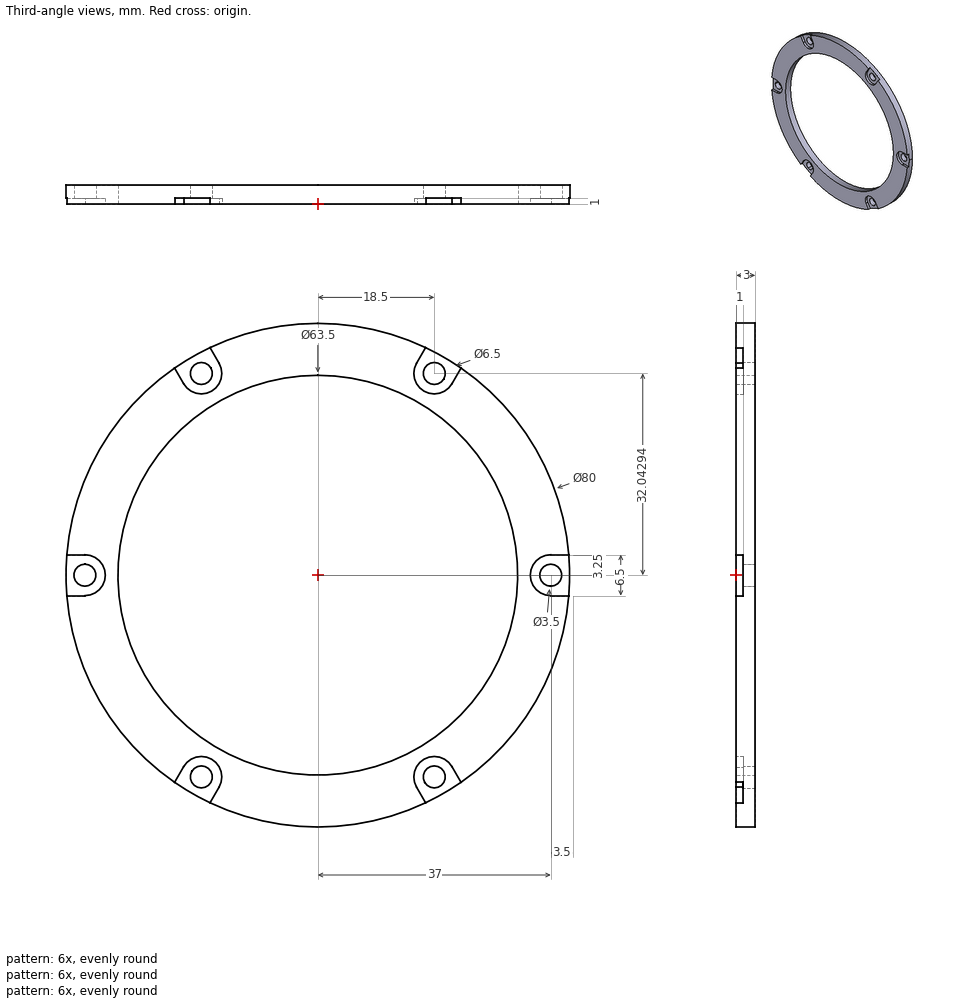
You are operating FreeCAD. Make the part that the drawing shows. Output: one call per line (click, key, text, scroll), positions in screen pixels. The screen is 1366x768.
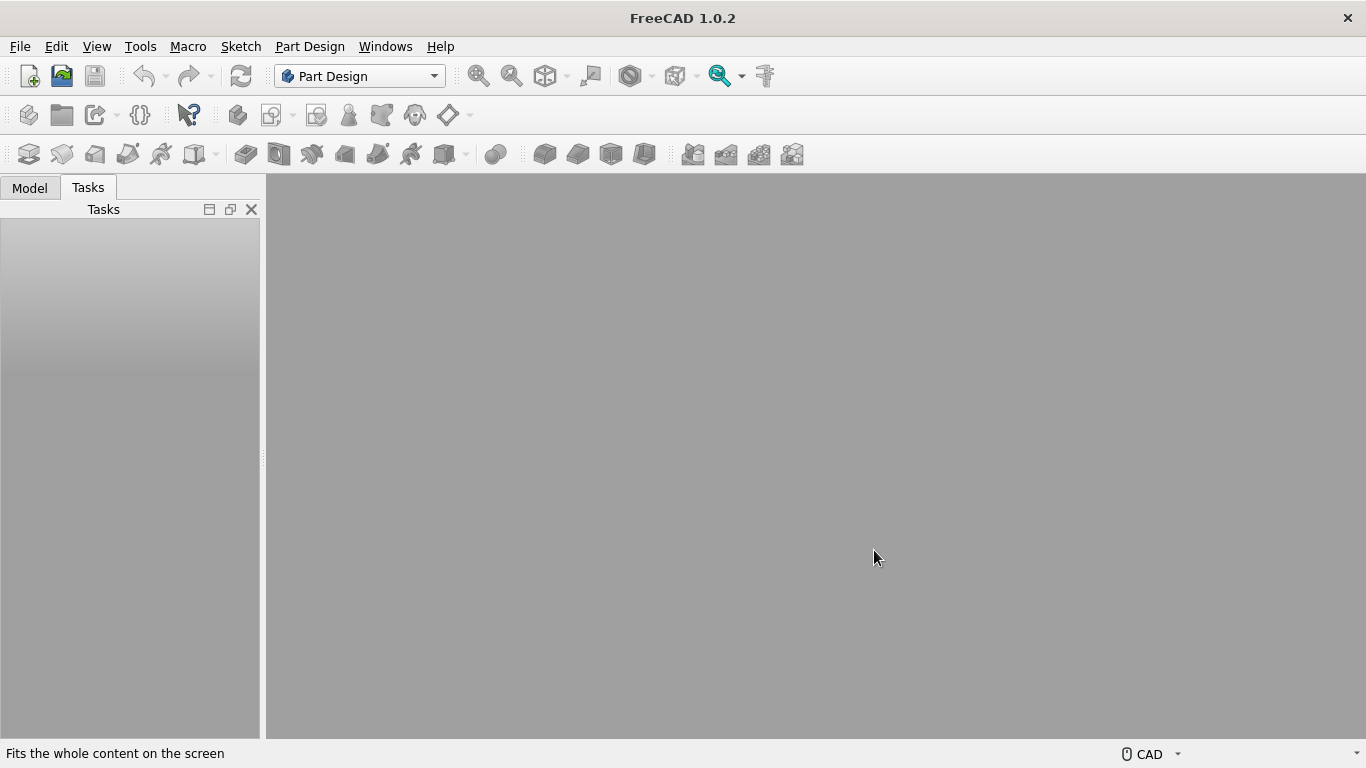
click(29, 76)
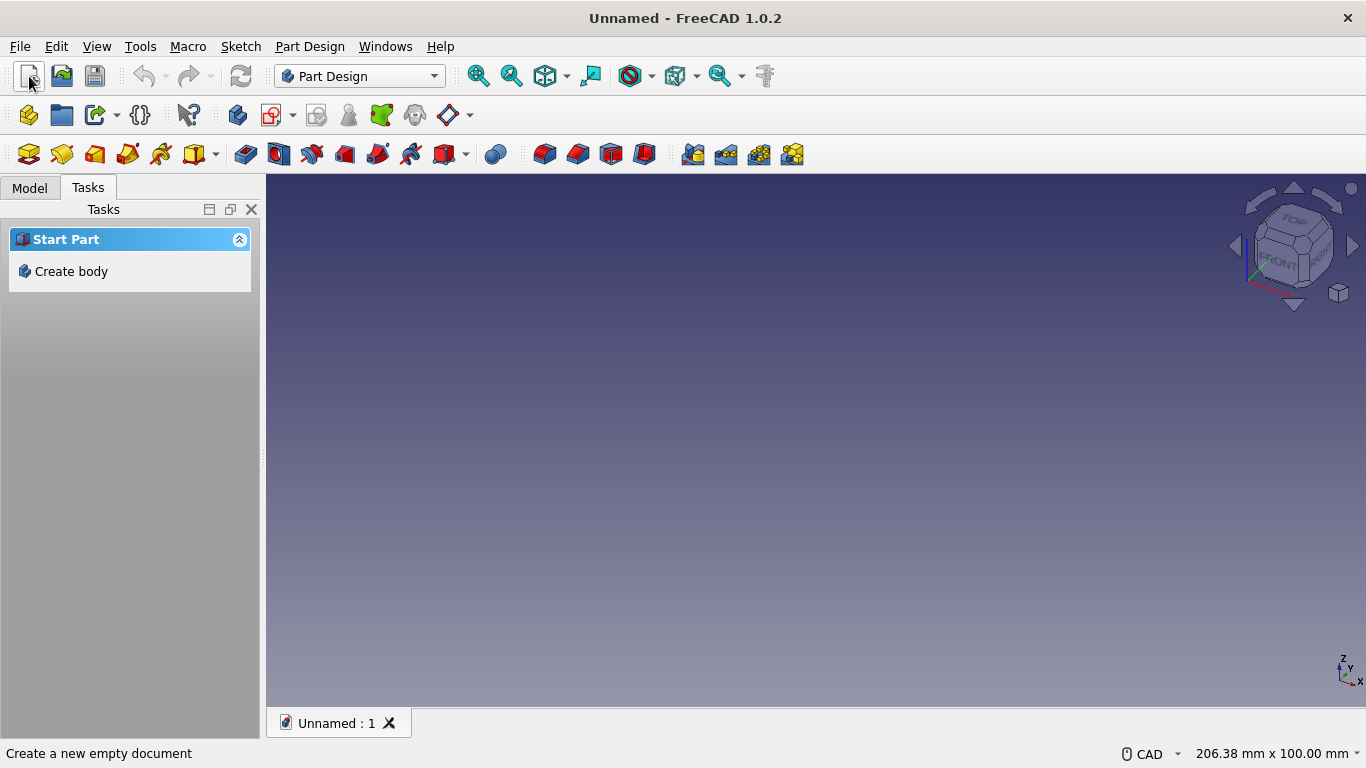
click(270, 116)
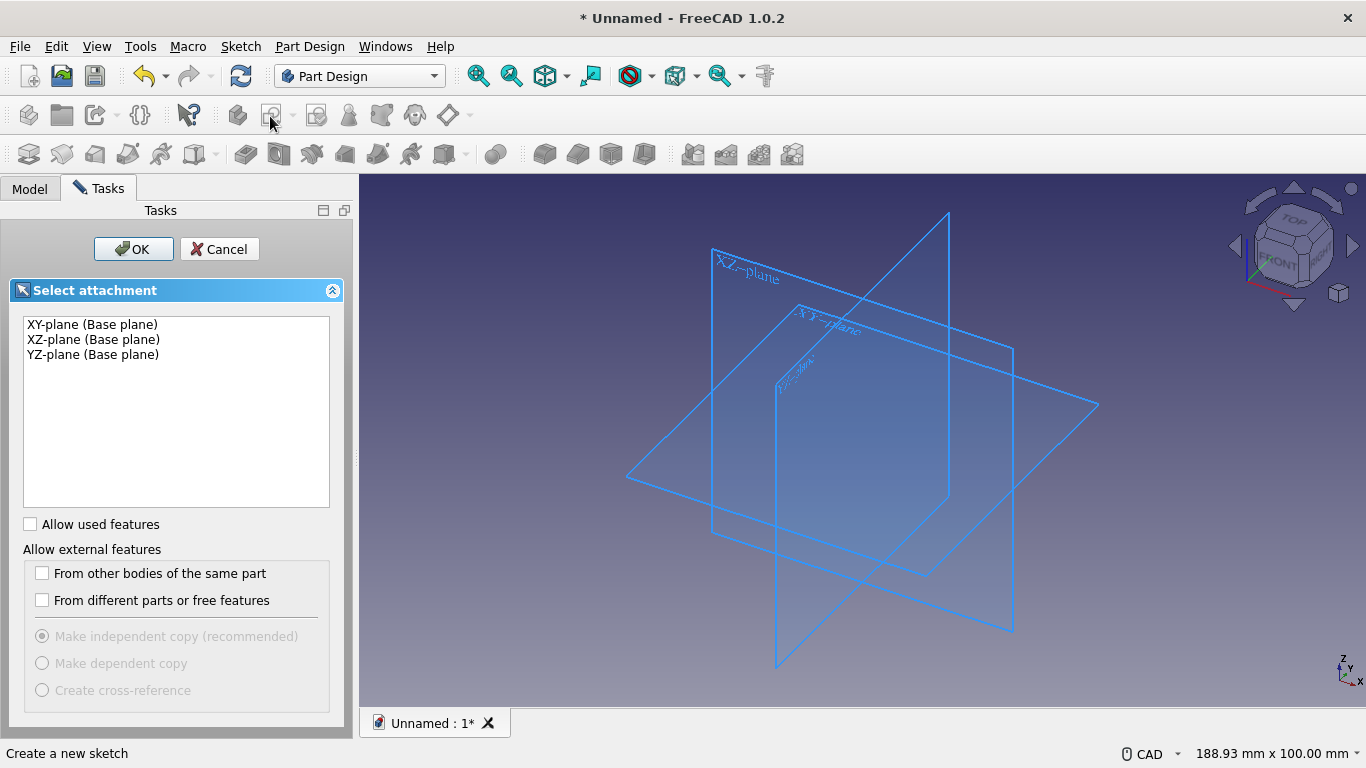
click(84, 340)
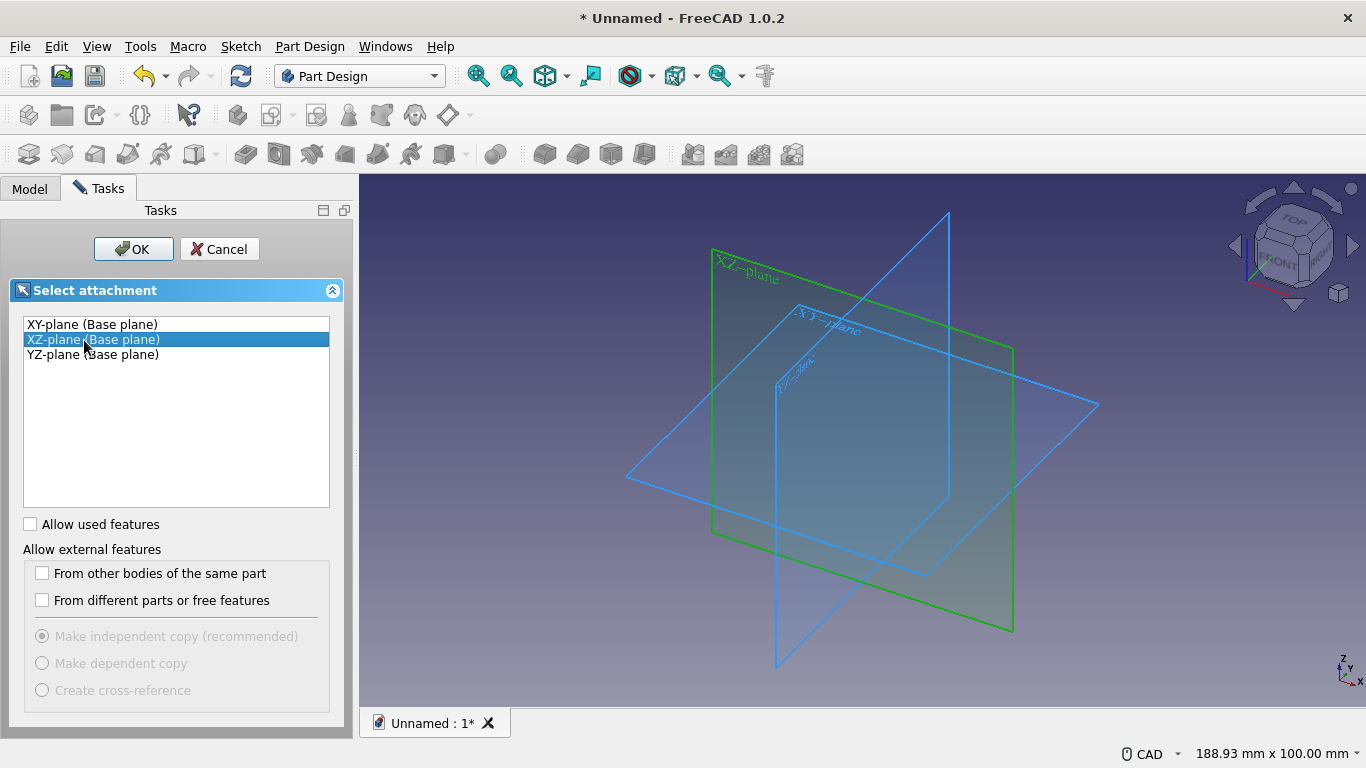
click(134, 249)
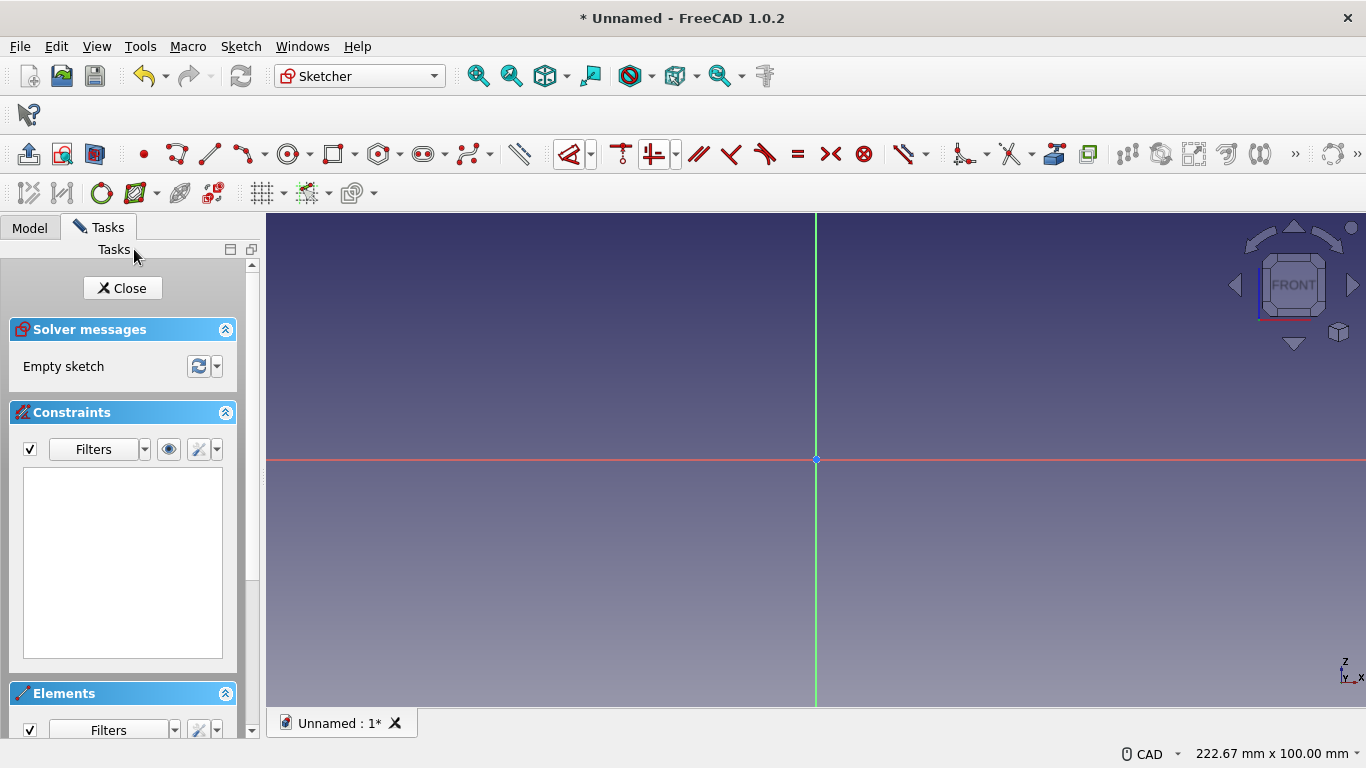
scroll(438, 460, down, 1)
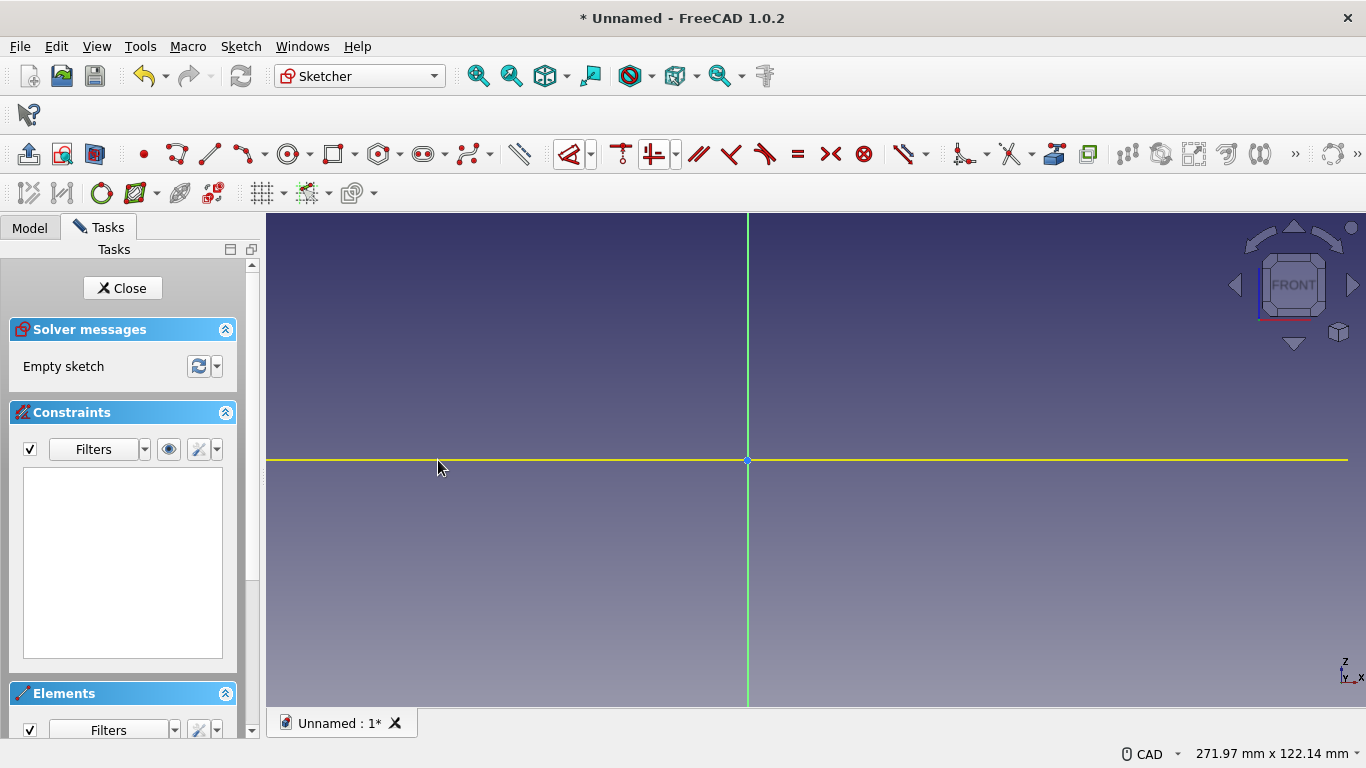
click(288, 154)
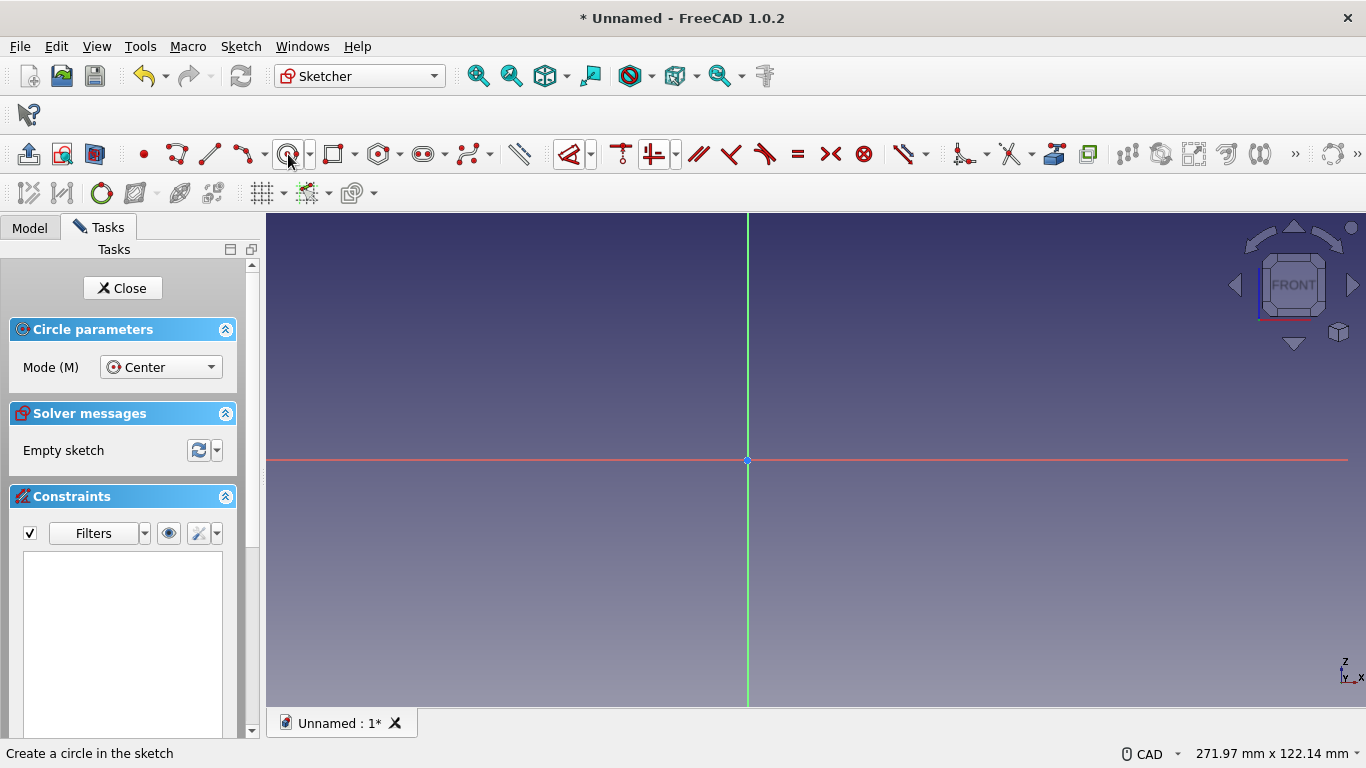
click(748, 460)
move(862, 346)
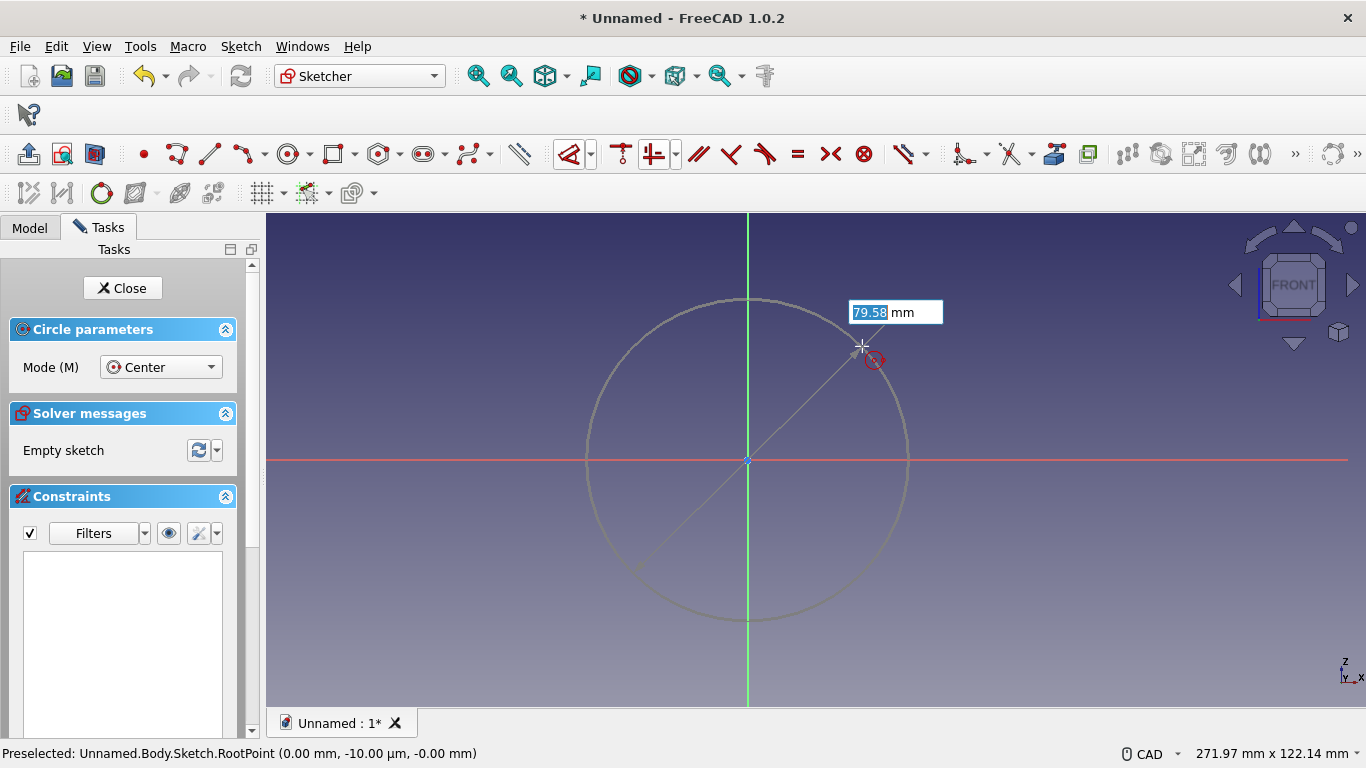
text(80)
key(Return)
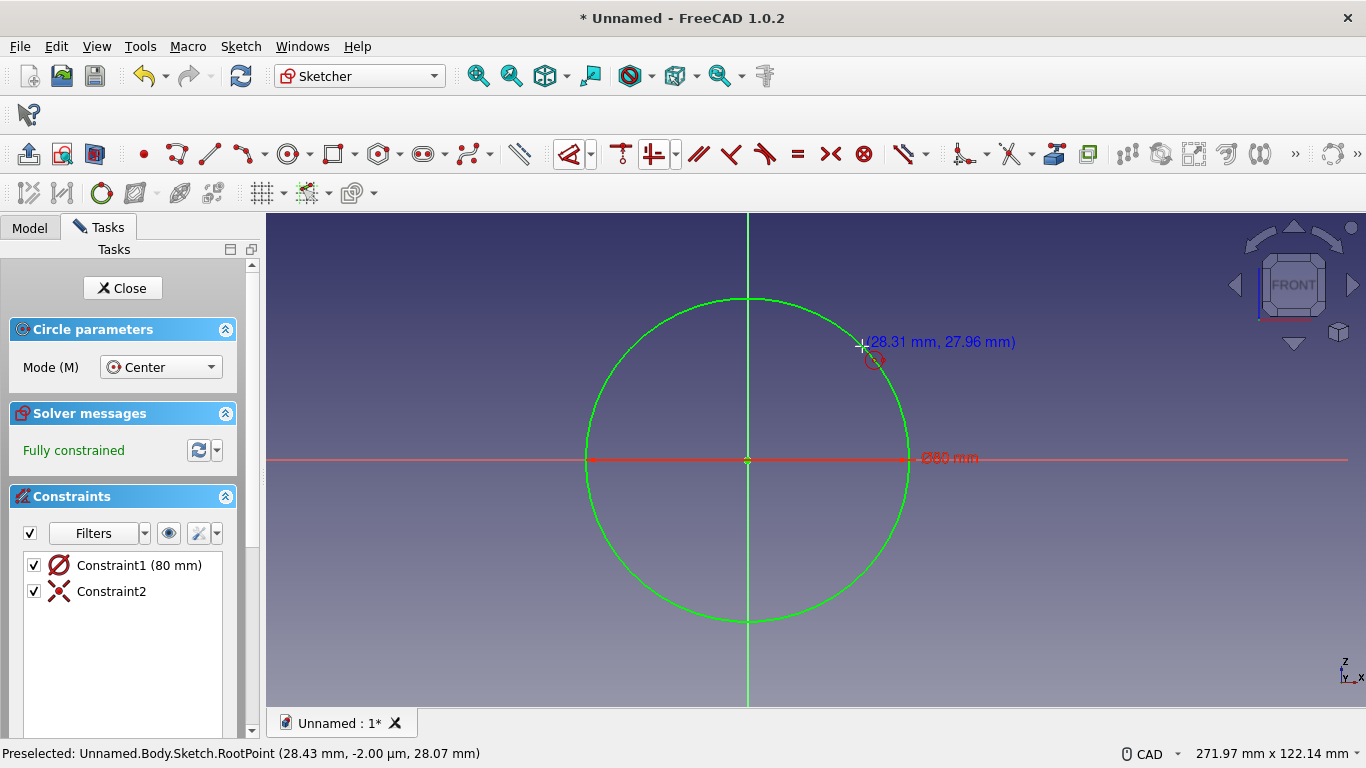
click(748, 460)
move(838, 369)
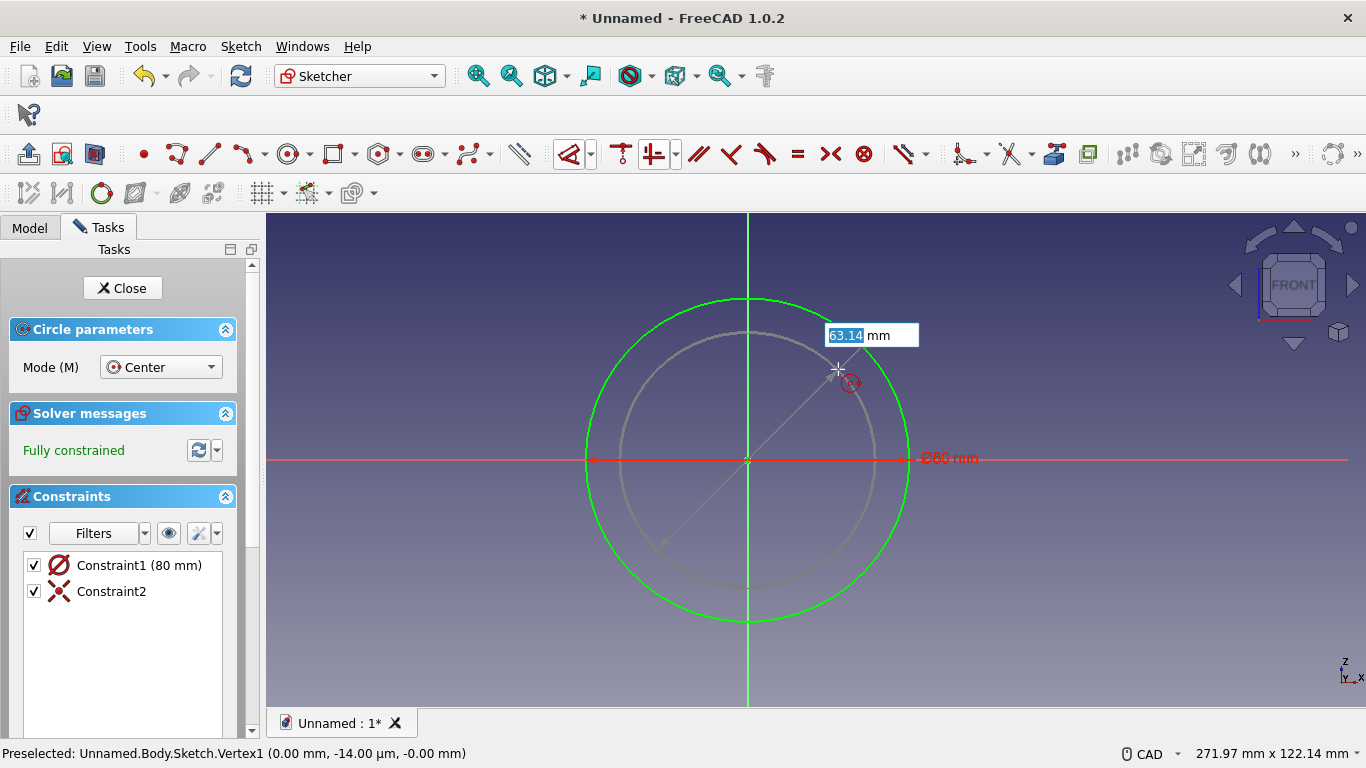
text(63.5)
key(Return)
key(Escape)